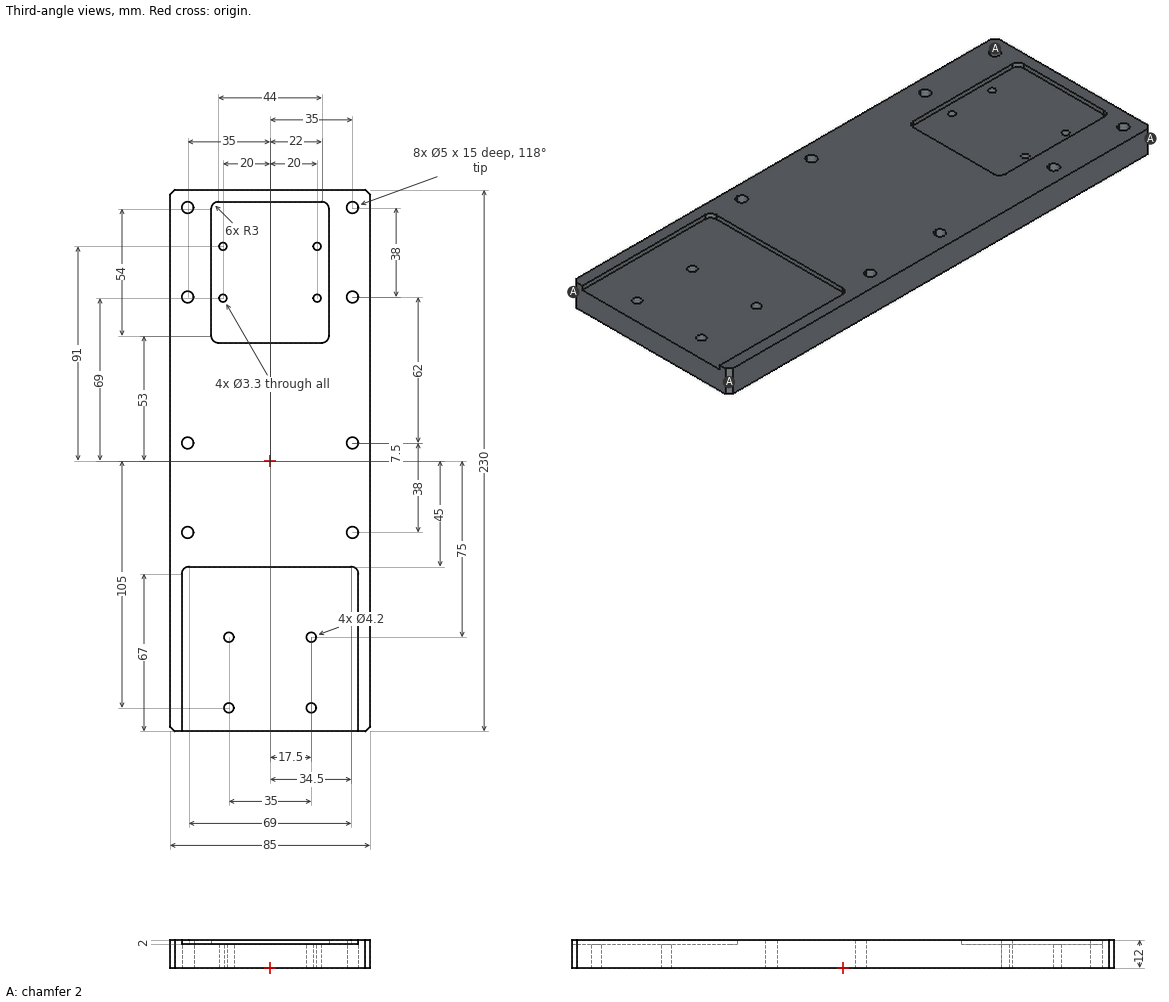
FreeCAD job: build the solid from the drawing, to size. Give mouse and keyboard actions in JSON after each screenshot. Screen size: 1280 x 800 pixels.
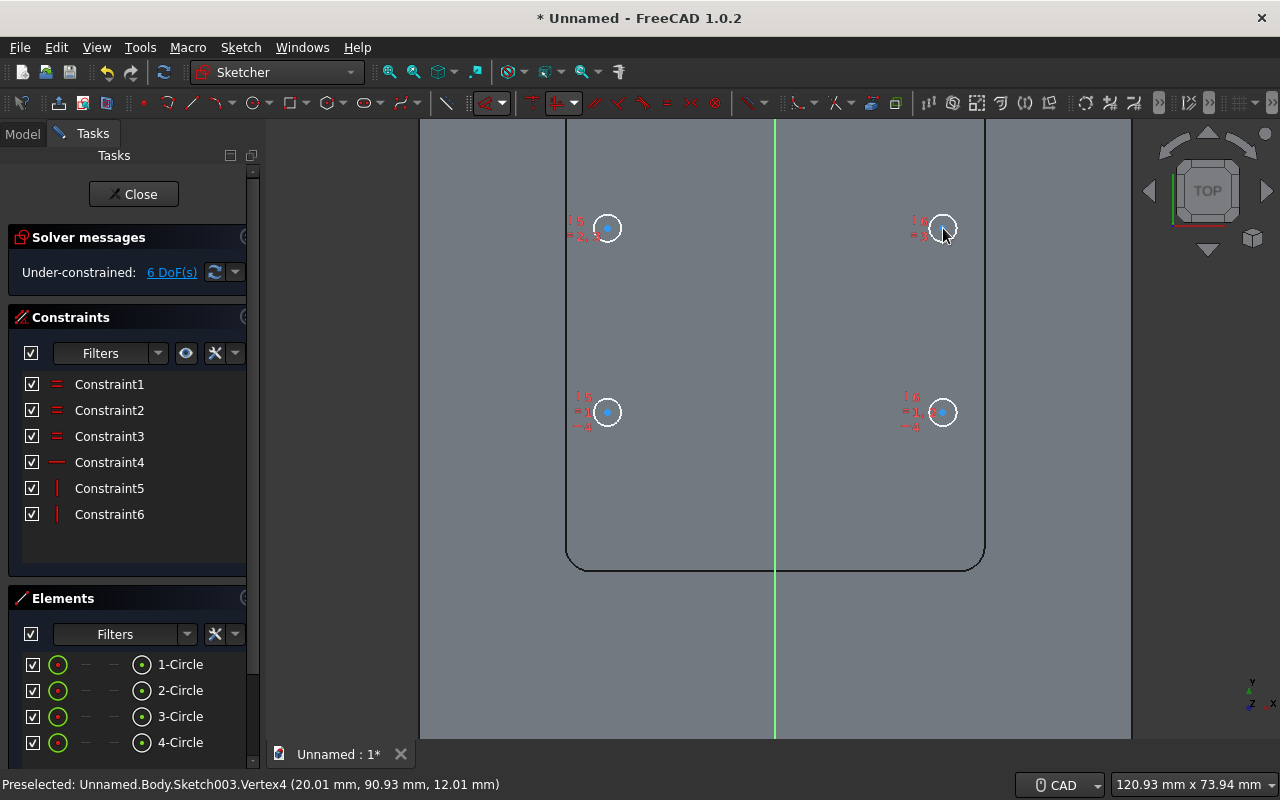
{"action": "left_click", "coordinate": [607, 228]}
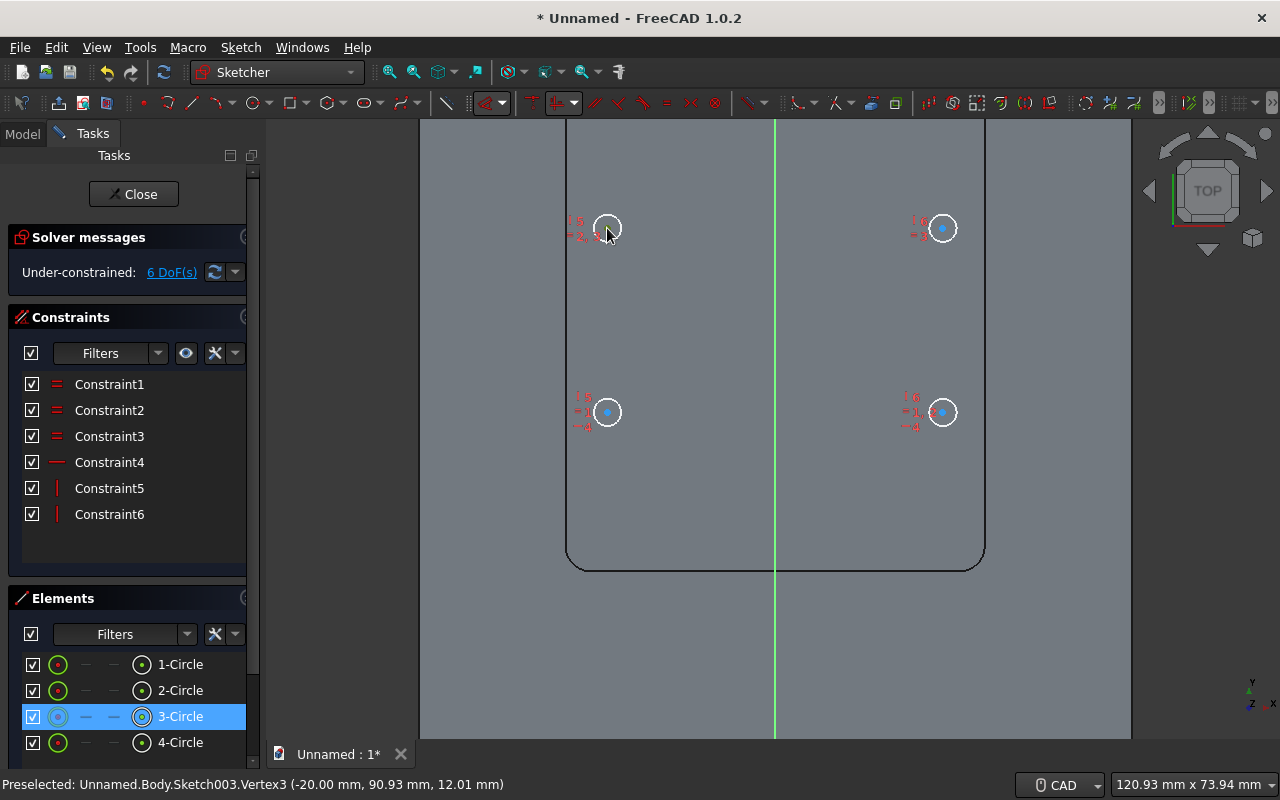
{"action": "left_click", "coordinate": [943, 228]}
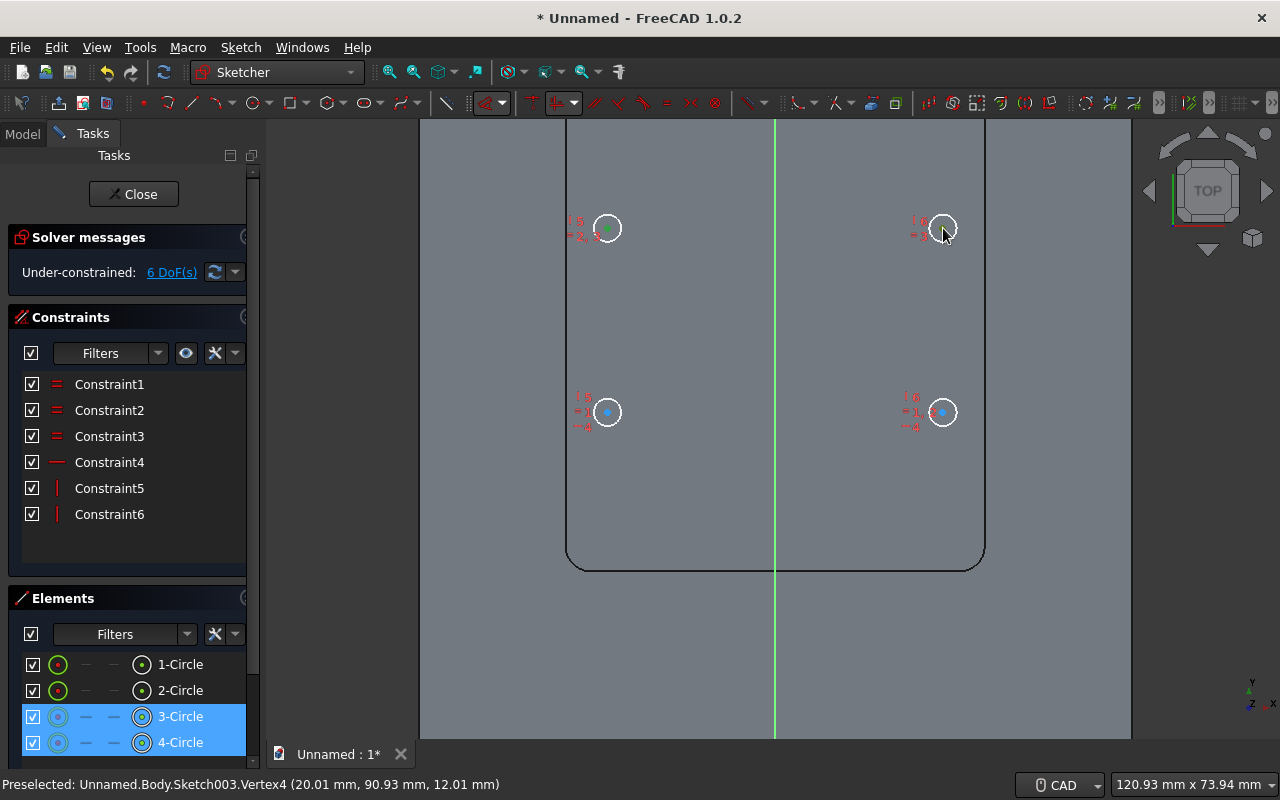
{"action": "key", "text": "h"}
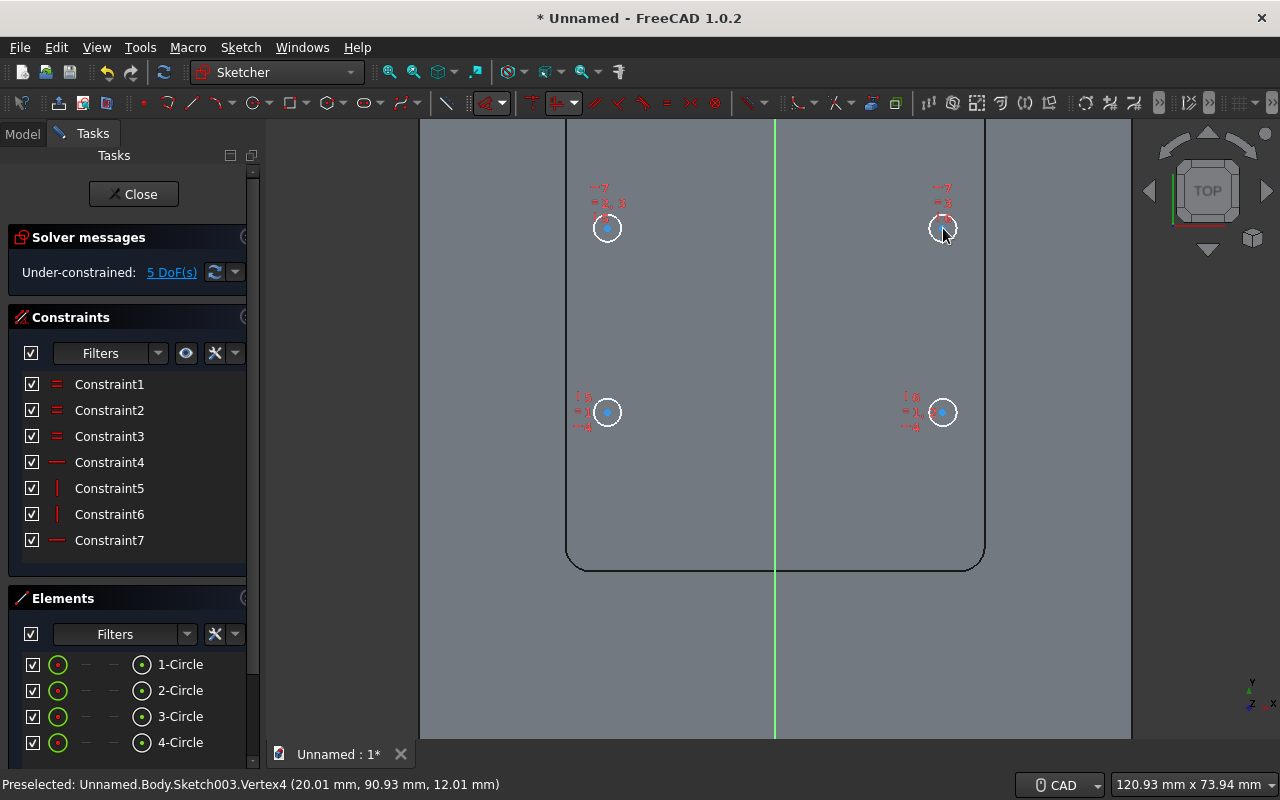
{"action": "scroll", "coordinate": [617, 403], "scroll_direction": "up", "scroll_amount": 2}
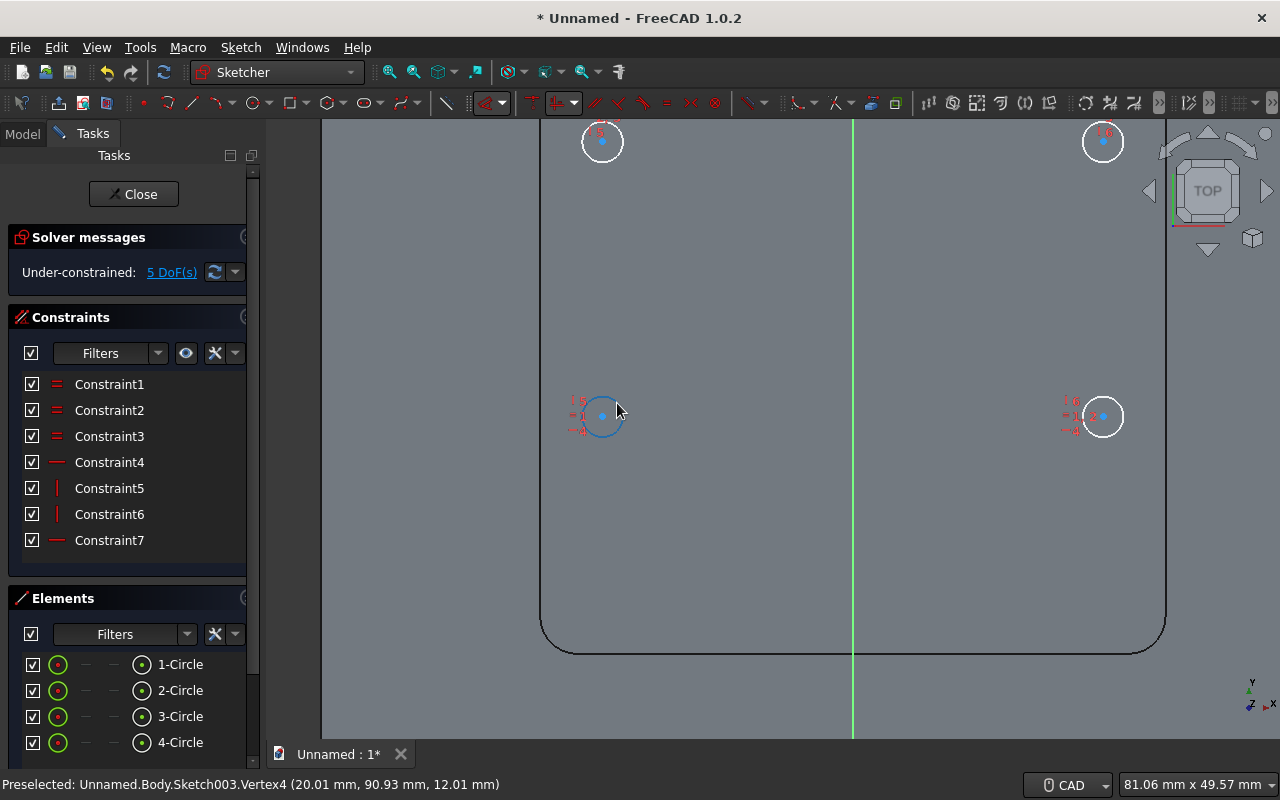
{"action": "left_click", "coordinate": [617, 402]}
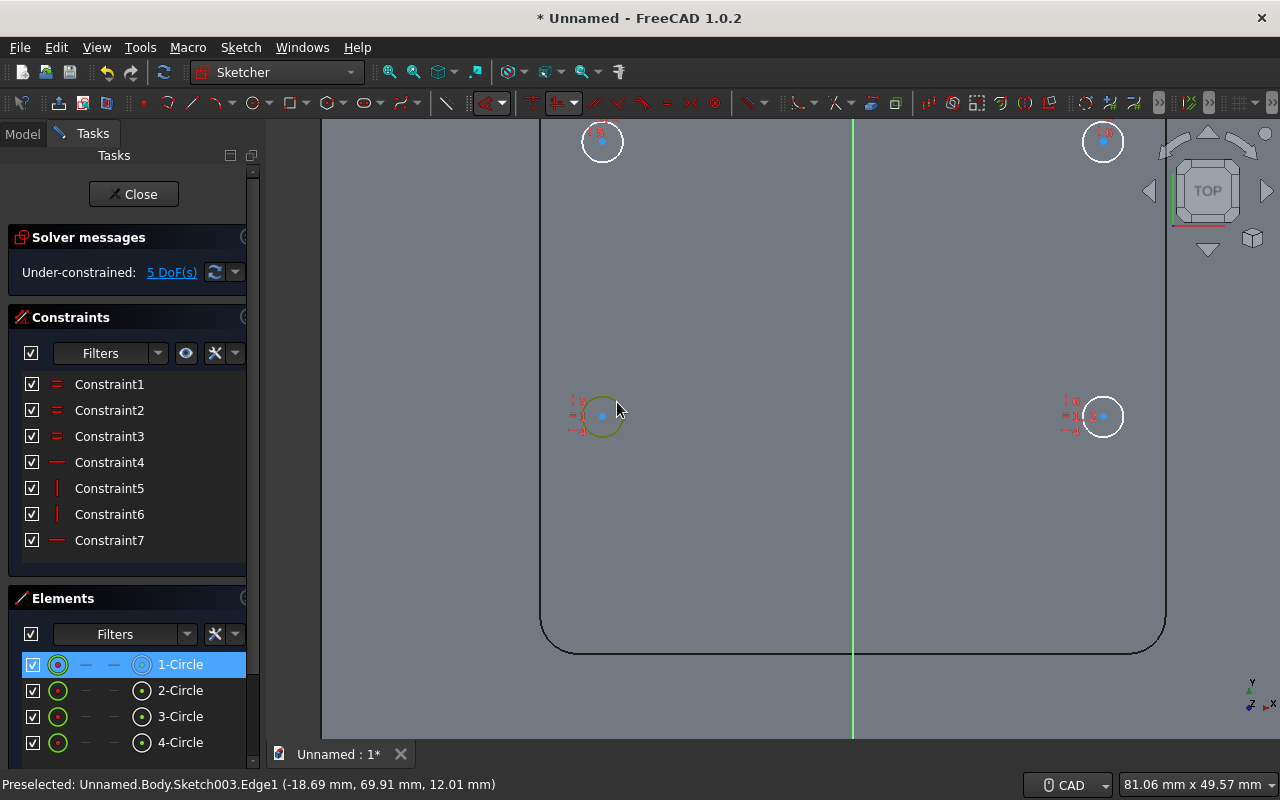
{"action": "key", "text": "k o"}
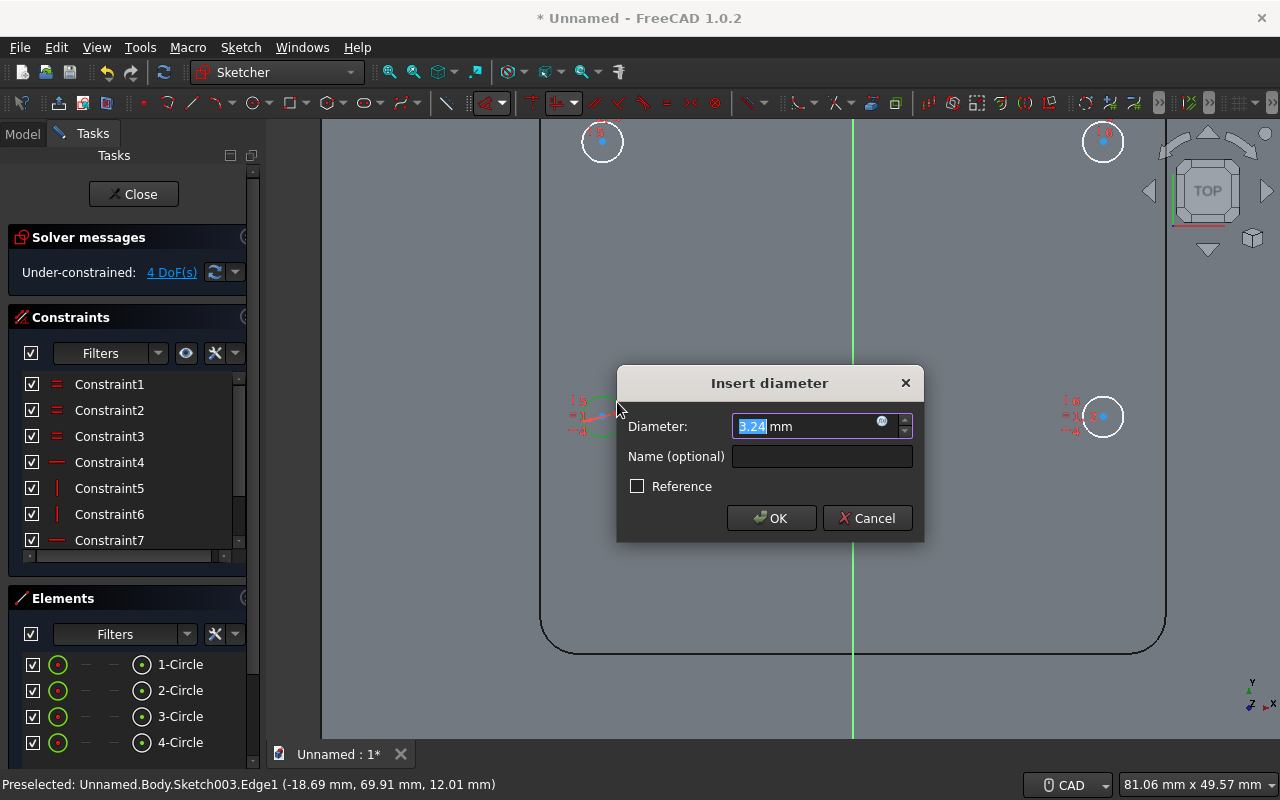
{"action": "type", "text": "3.3"}
{"action": "key", "text": "Return"}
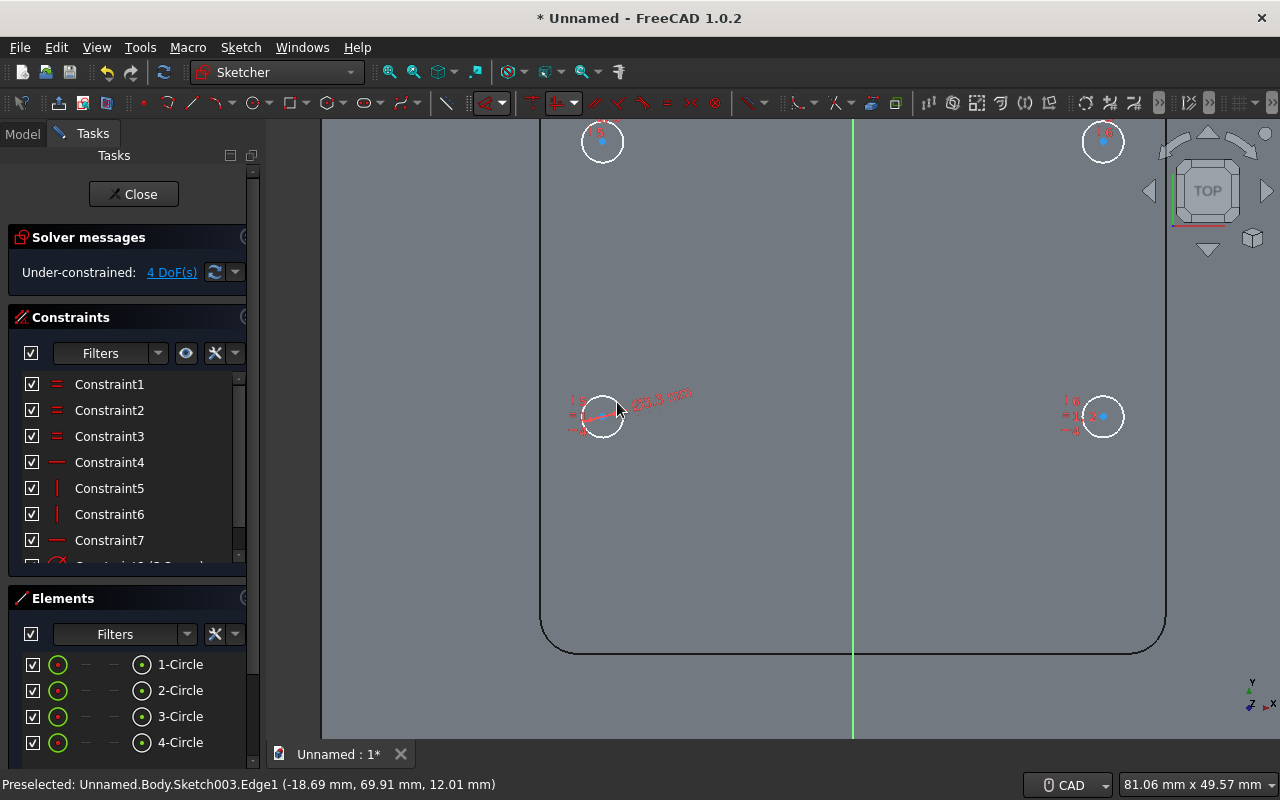
{"action": "left_click", "coordinate": [603, 417]}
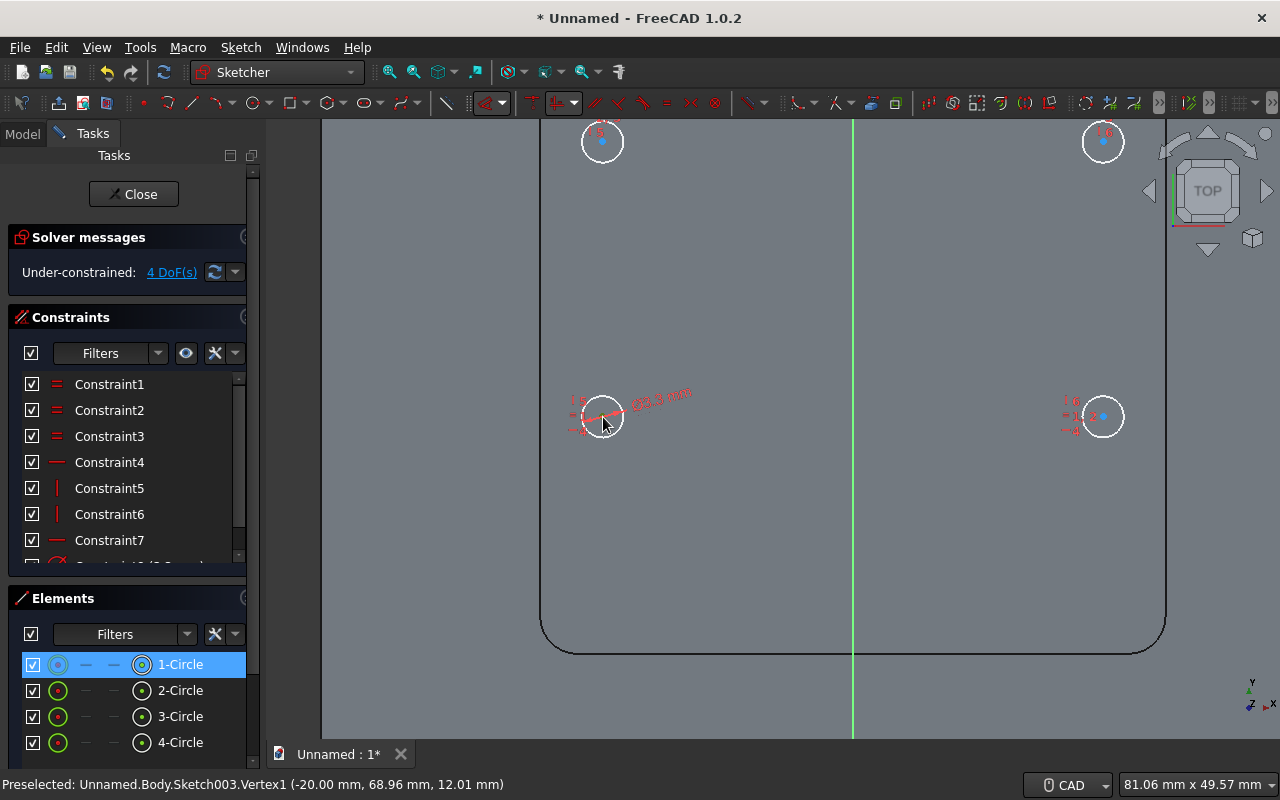
{"action": "key", "text": "l"}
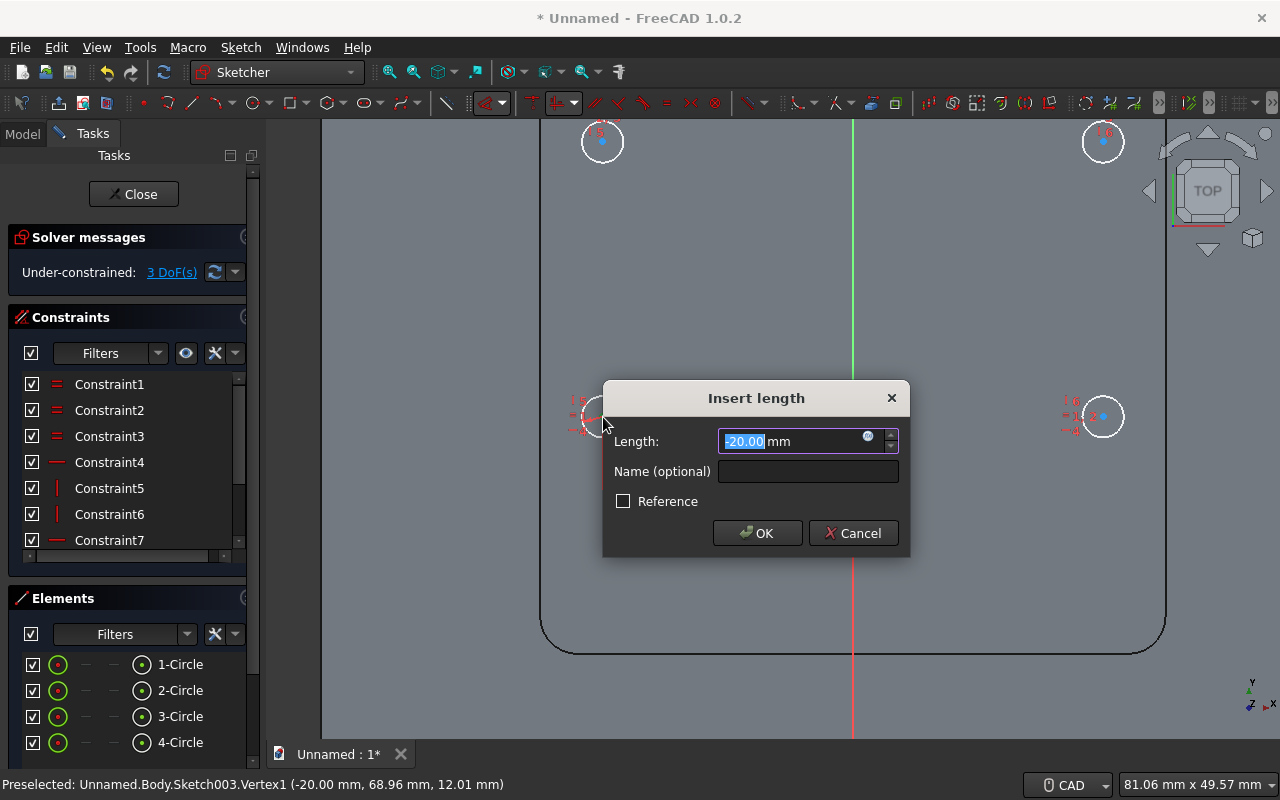
{"action": "type", "text": "-20"}
{"action": "key", "text": "Return"}